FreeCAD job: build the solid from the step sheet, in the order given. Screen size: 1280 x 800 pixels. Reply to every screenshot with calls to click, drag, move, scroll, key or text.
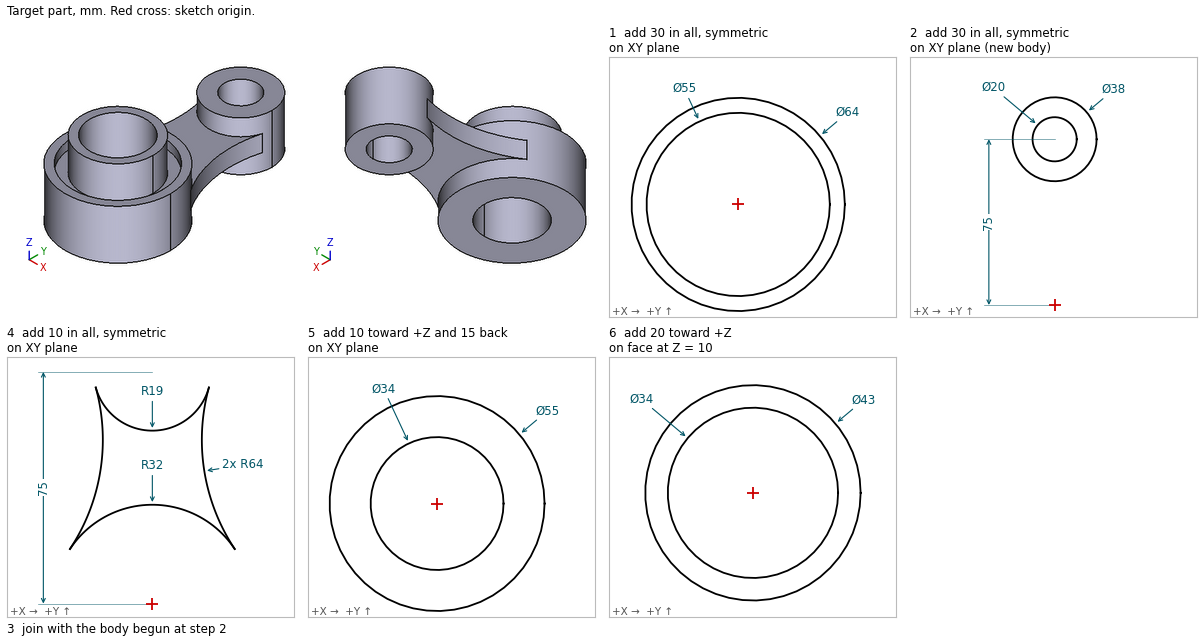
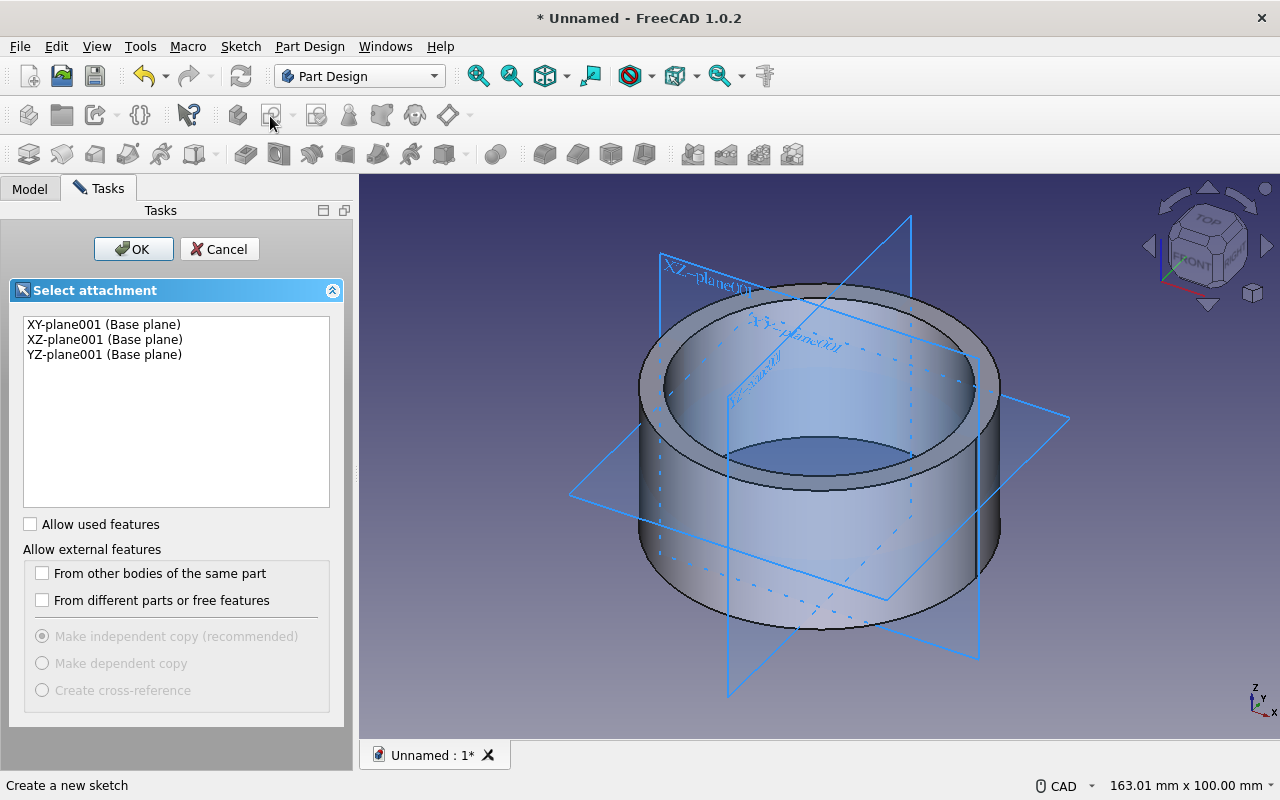
click(84, 324)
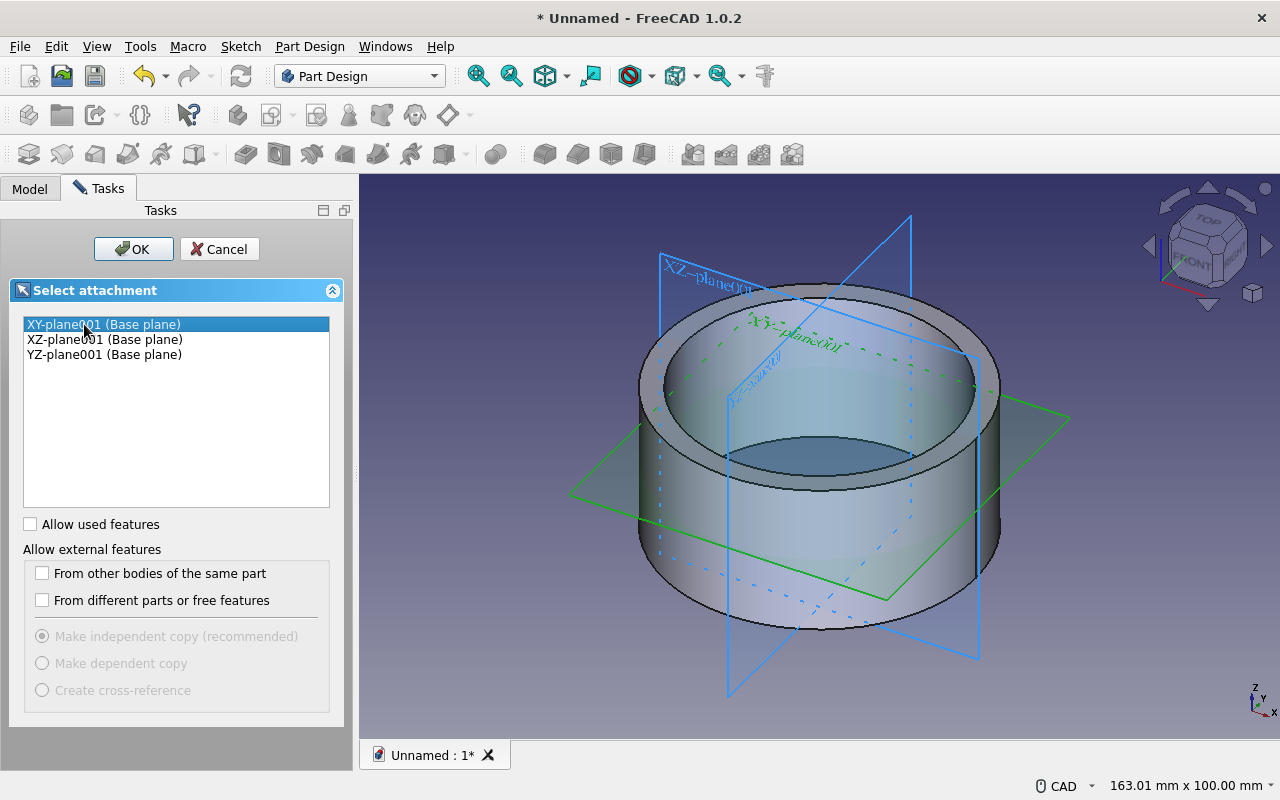
click(134, 249)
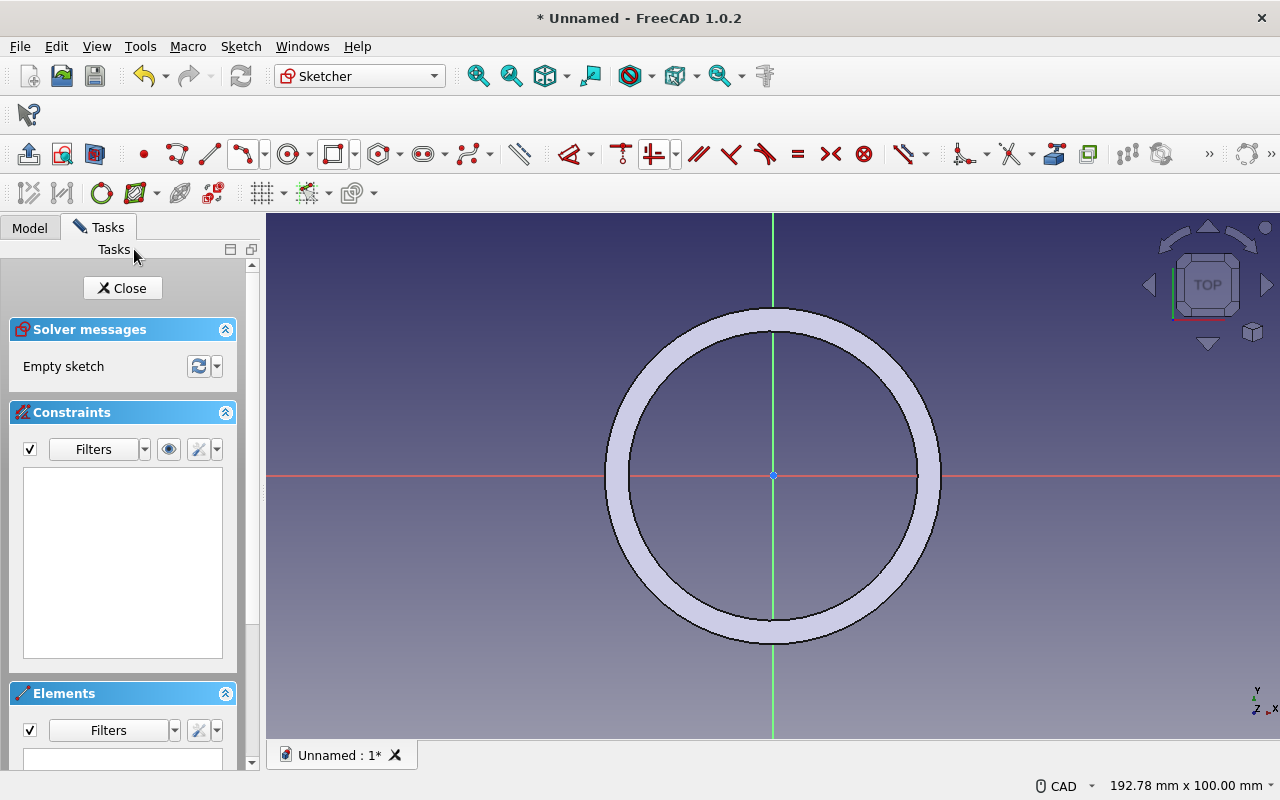
scroll(621, 711, down, 3)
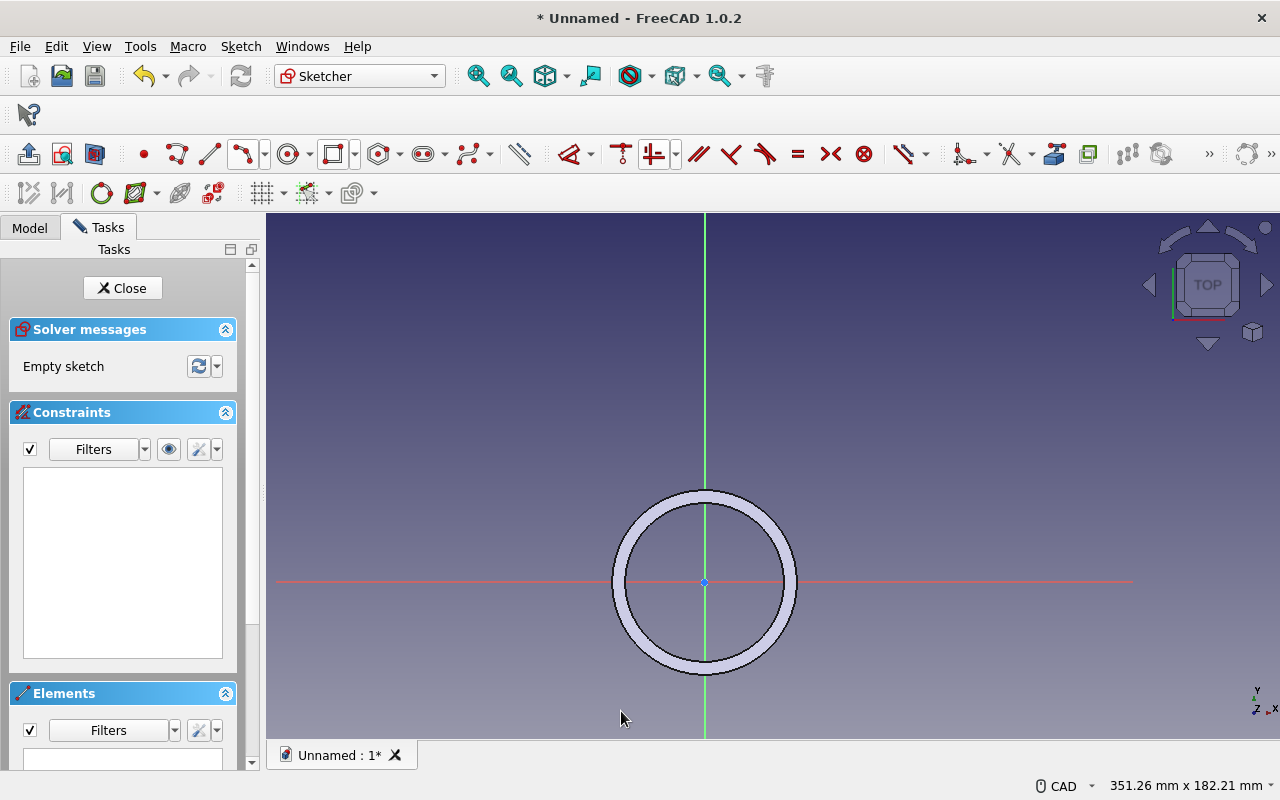
click(288, 154)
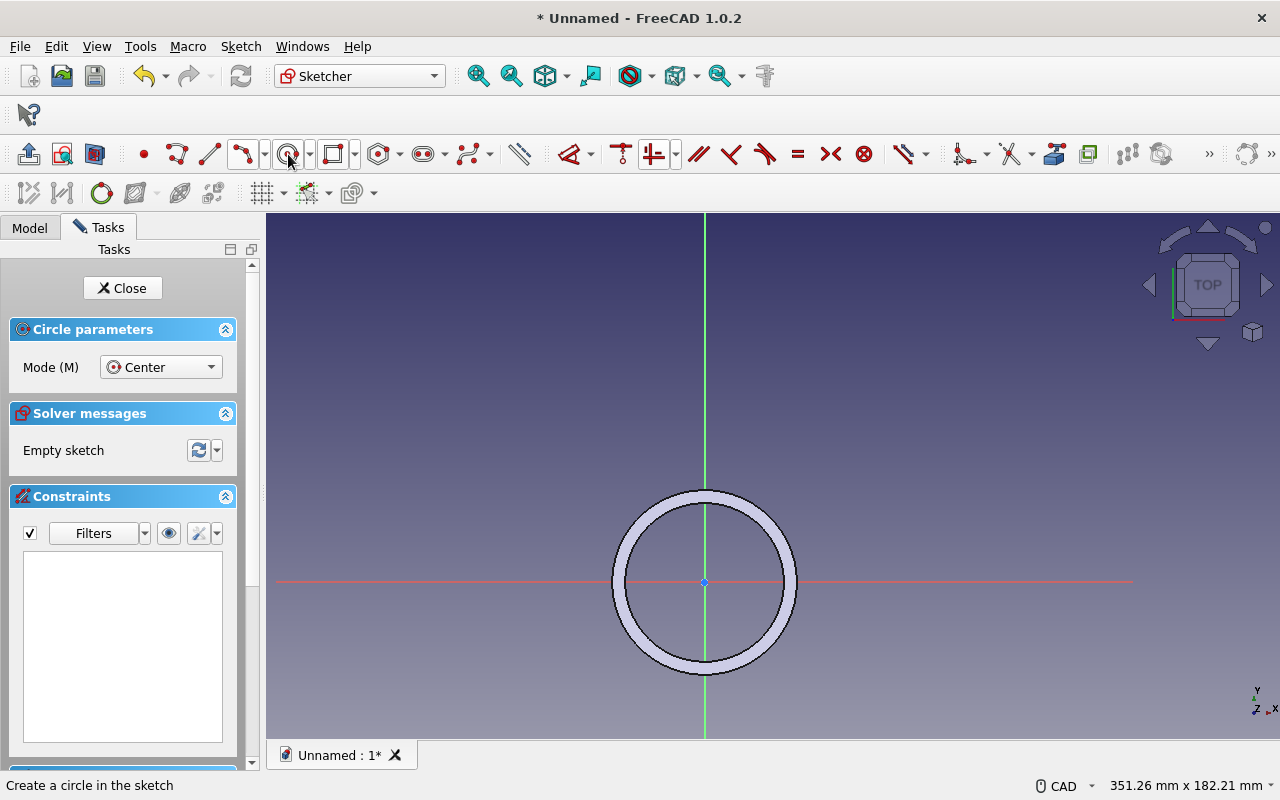
click(705, 366)
click(743, 327)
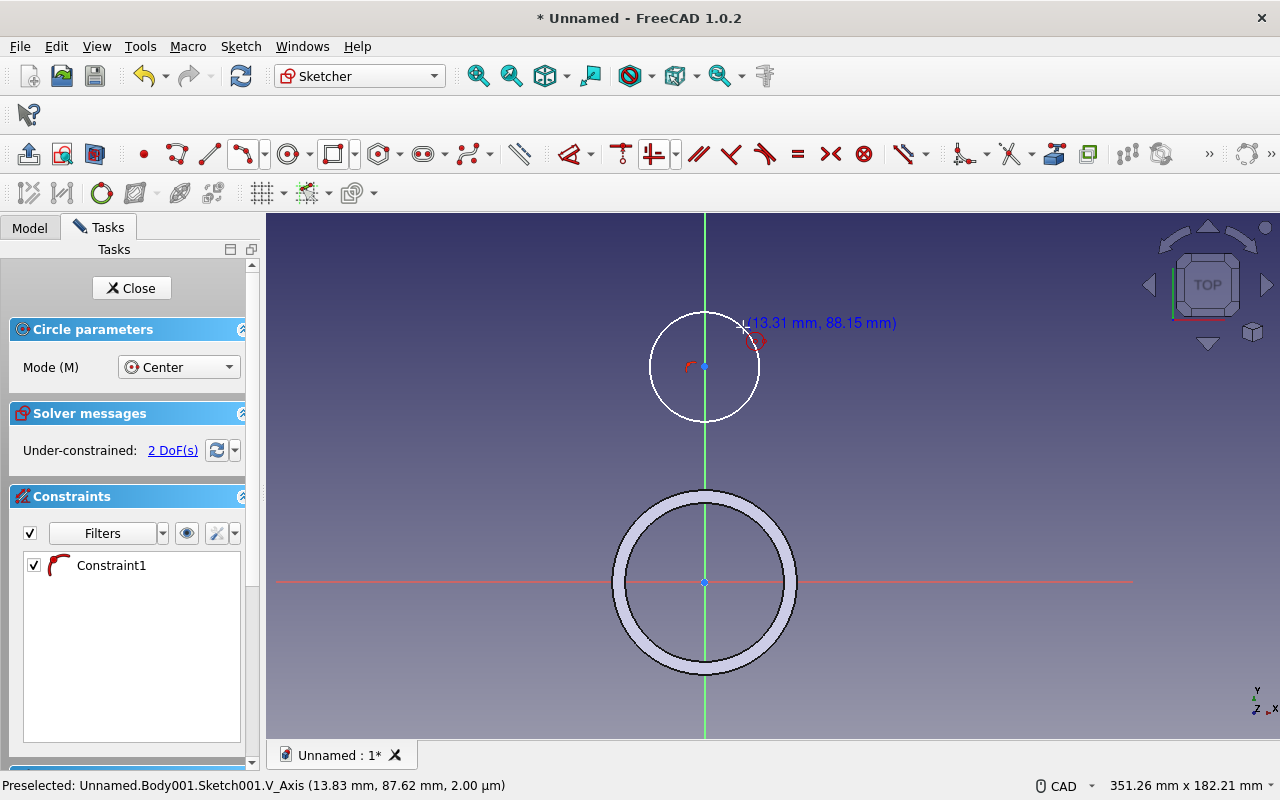
click(705, 367)
click(725, 346)
key(Escape)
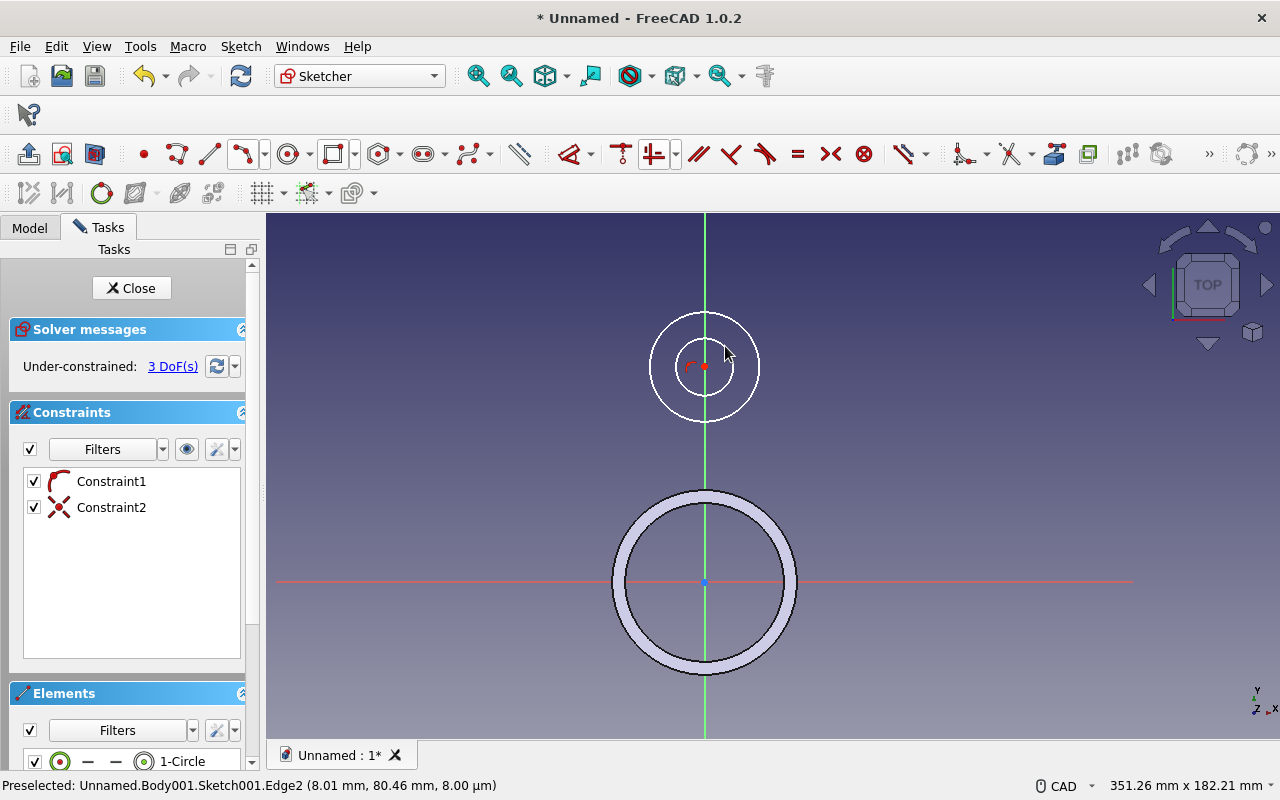
key(d)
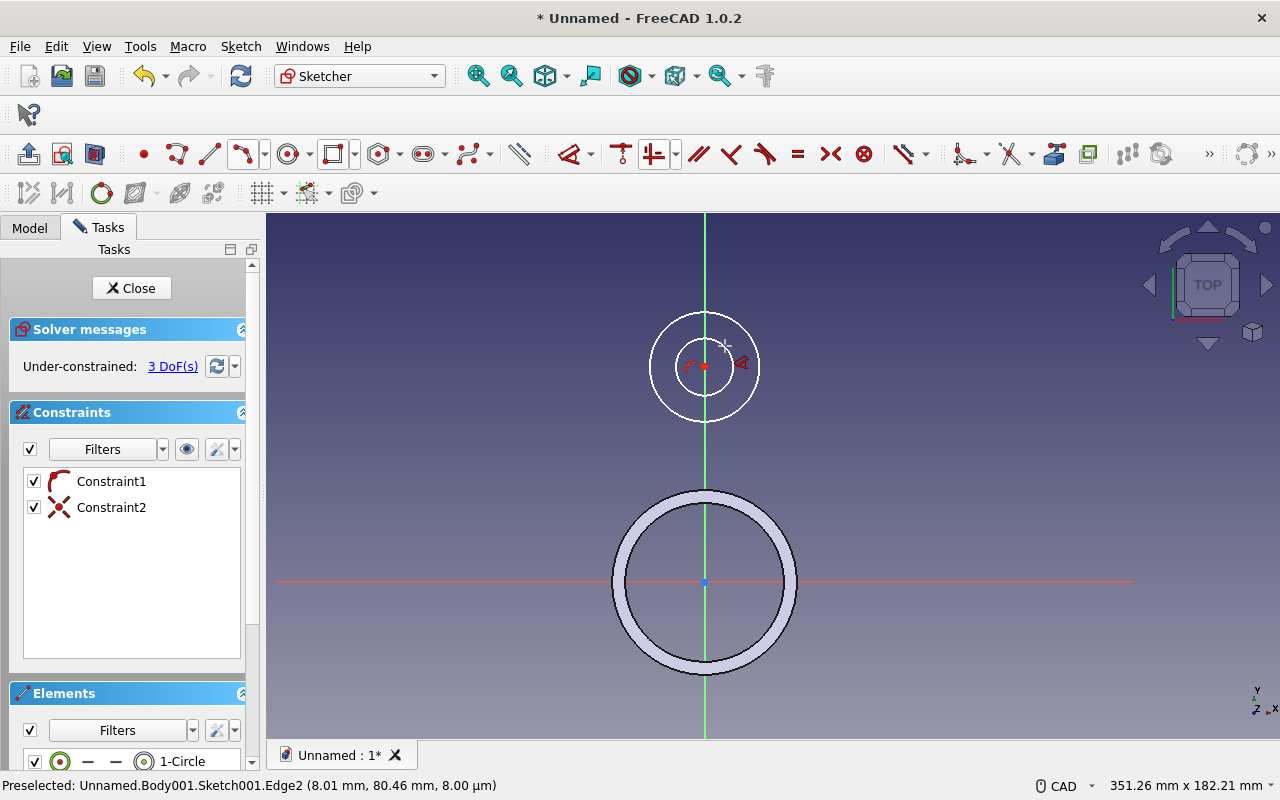
click(743, 328)
click(765, 305)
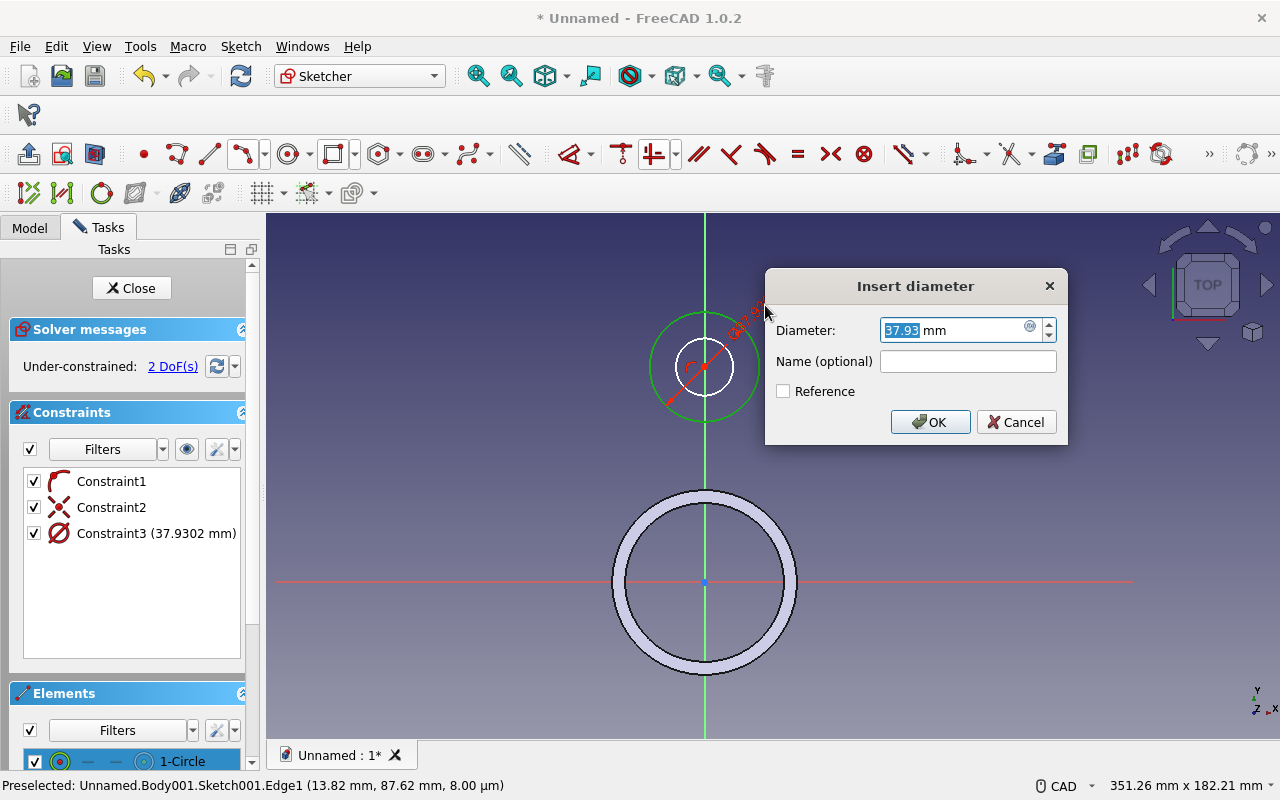
text(38)
key(Return)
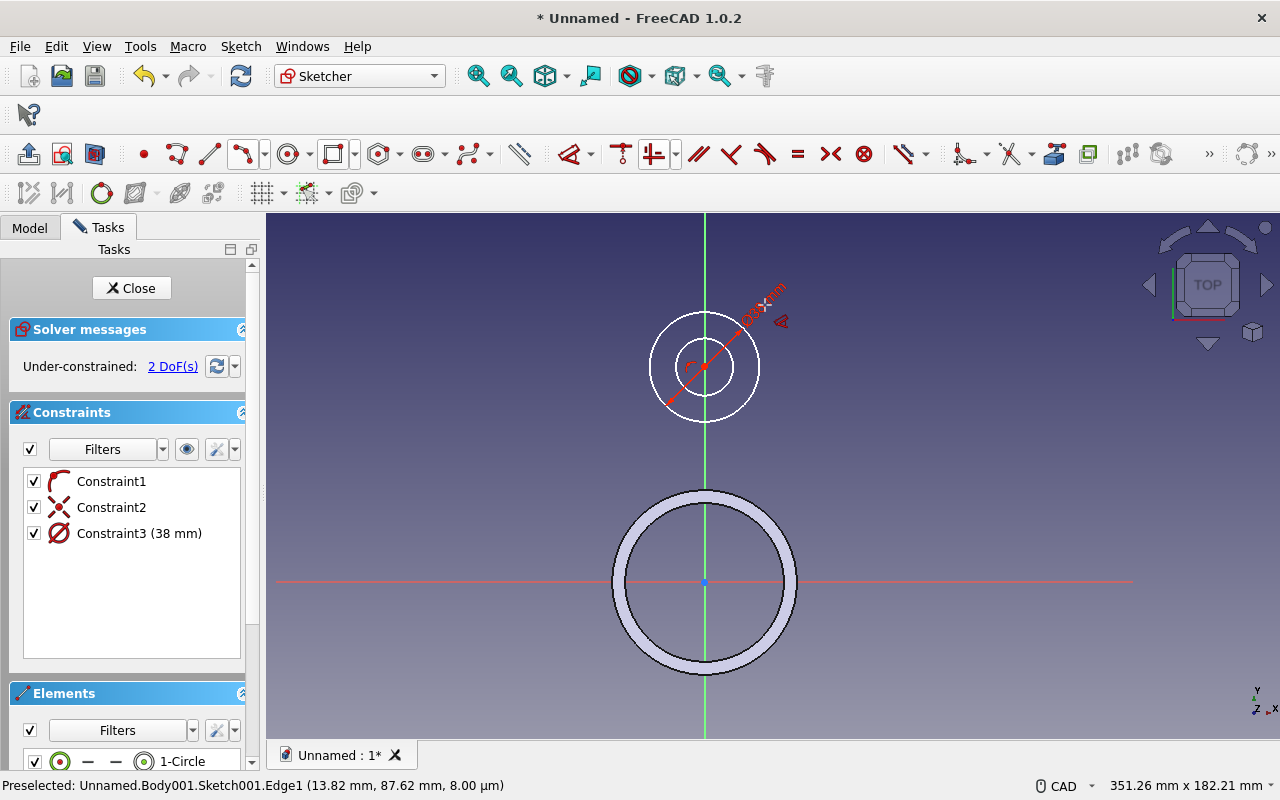
click(725, 347)
click(785, 344)